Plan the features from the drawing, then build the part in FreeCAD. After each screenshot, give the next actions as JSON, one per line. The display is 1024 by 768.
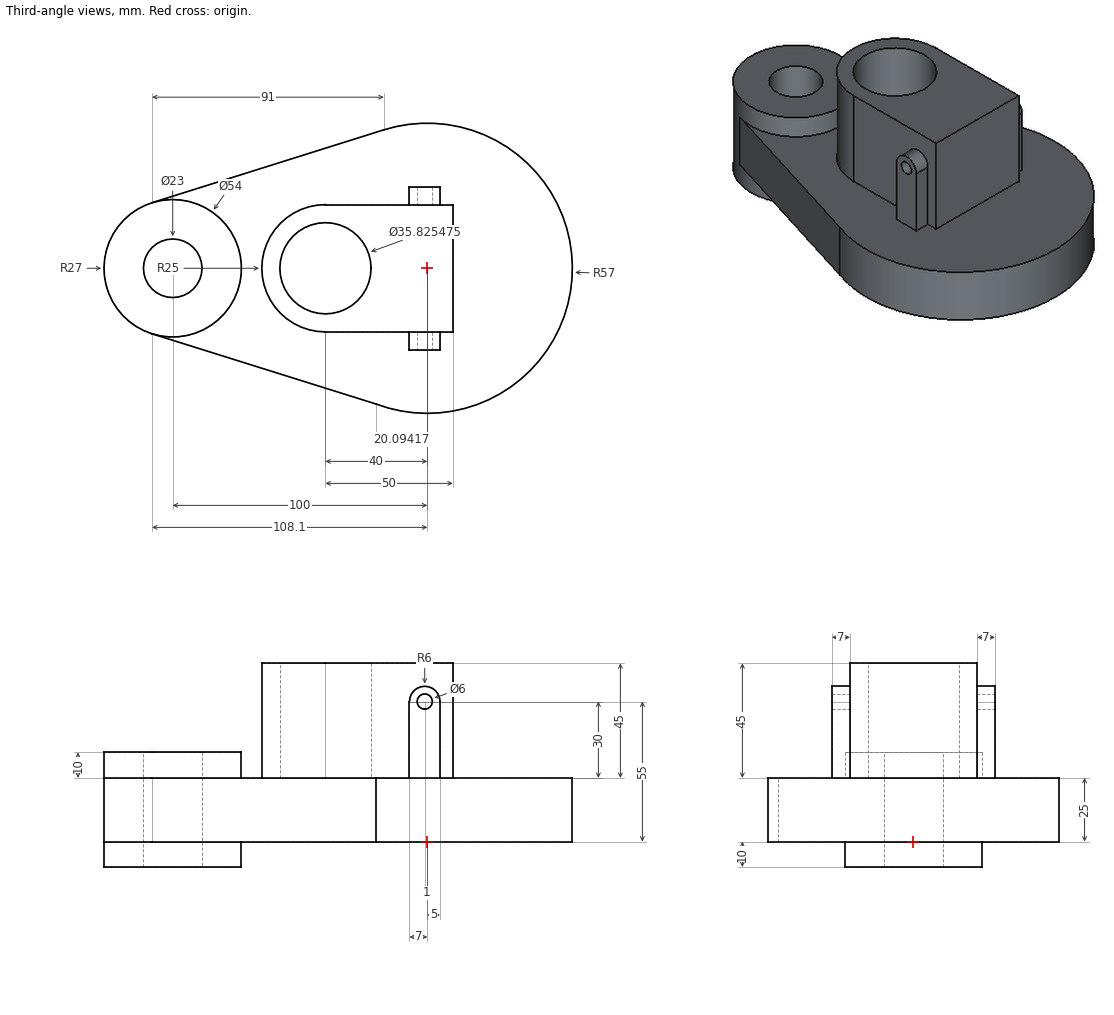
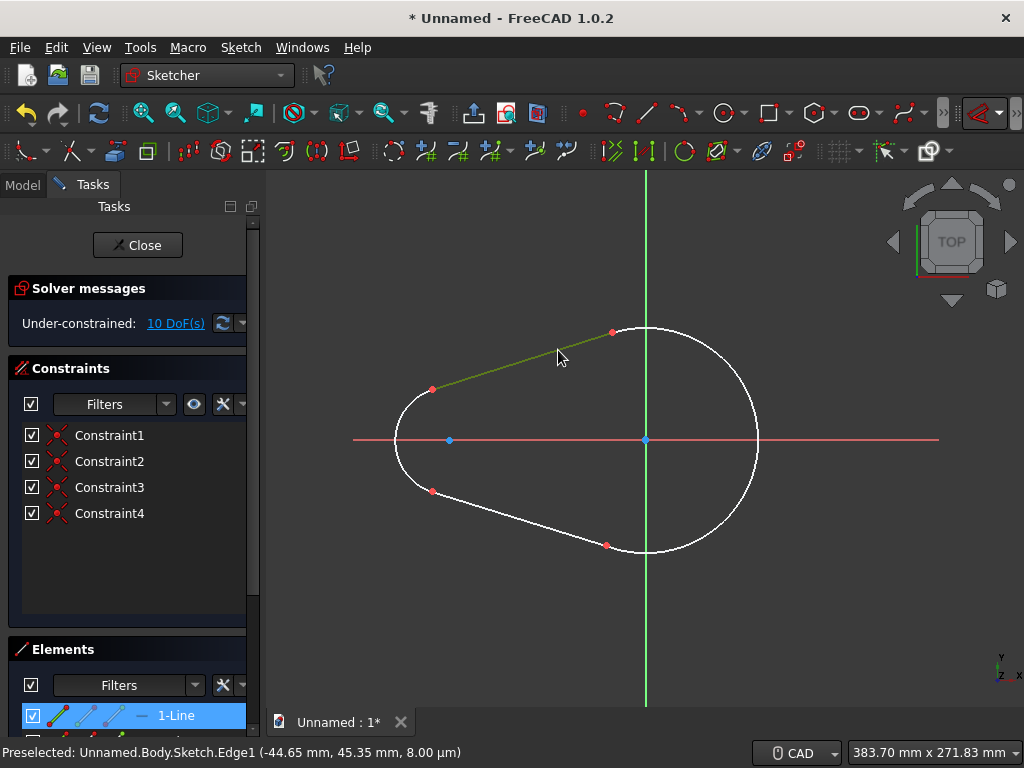
{"action": "left_click", "coordinate": [402, 415]}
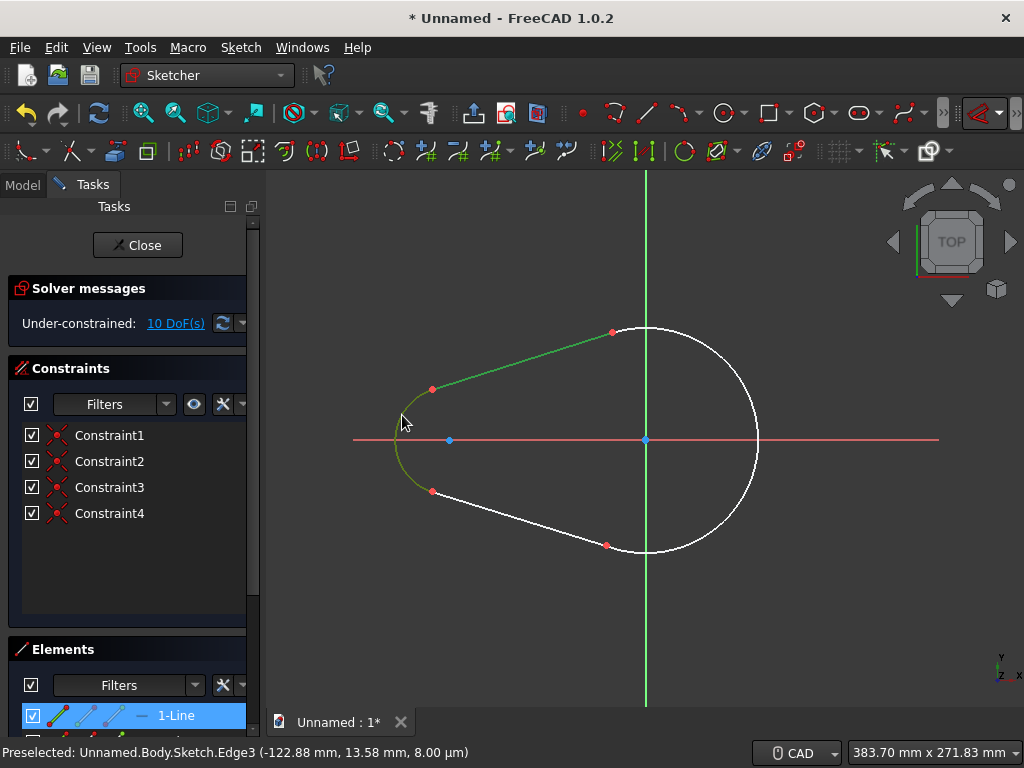
{"action": "key", "text": "t"}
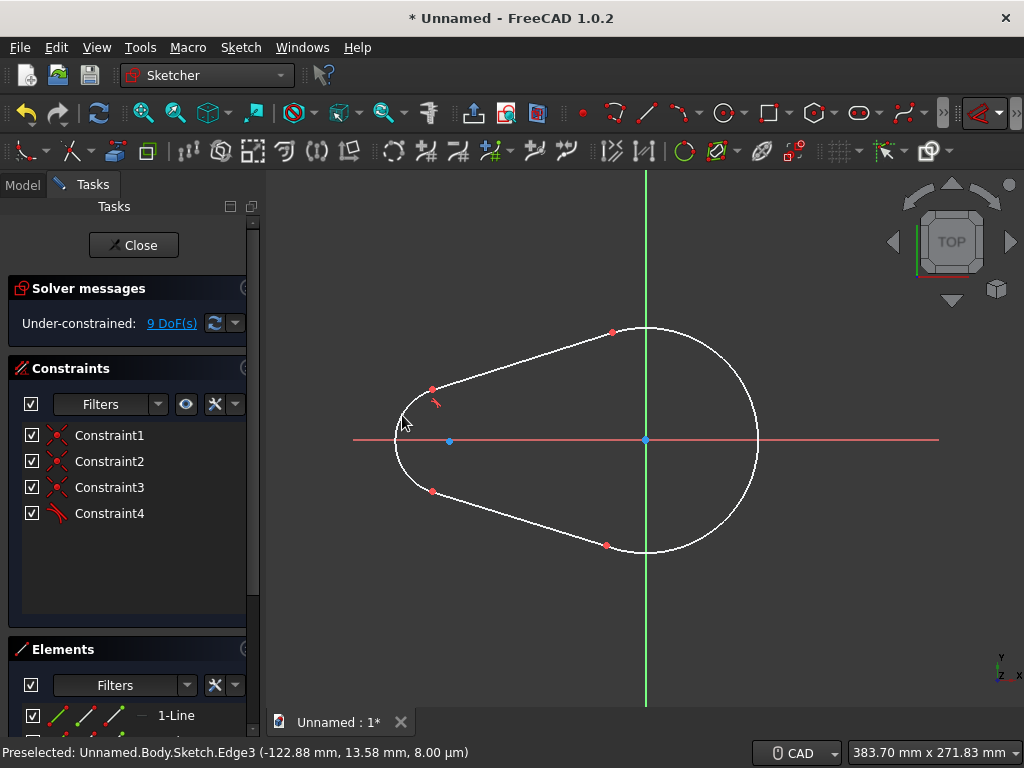
{"action": "left_click_drag", "start_coordinate": [636, 430], "coordinate": [656, 451]}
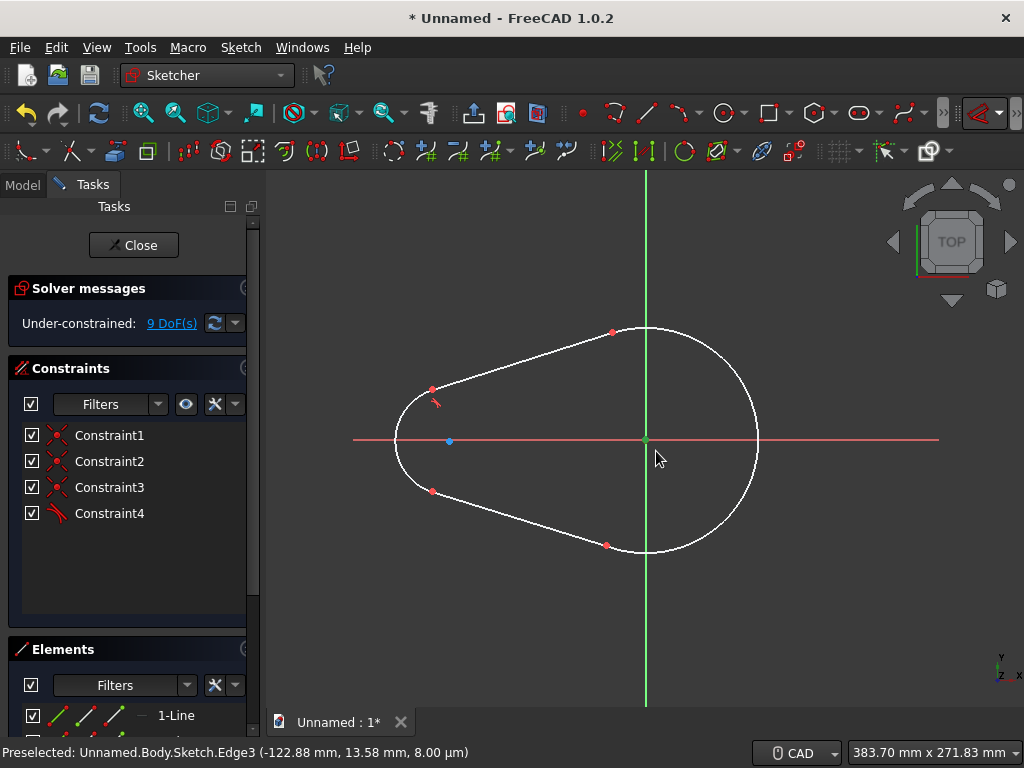
{"action": "key", "text": "c"}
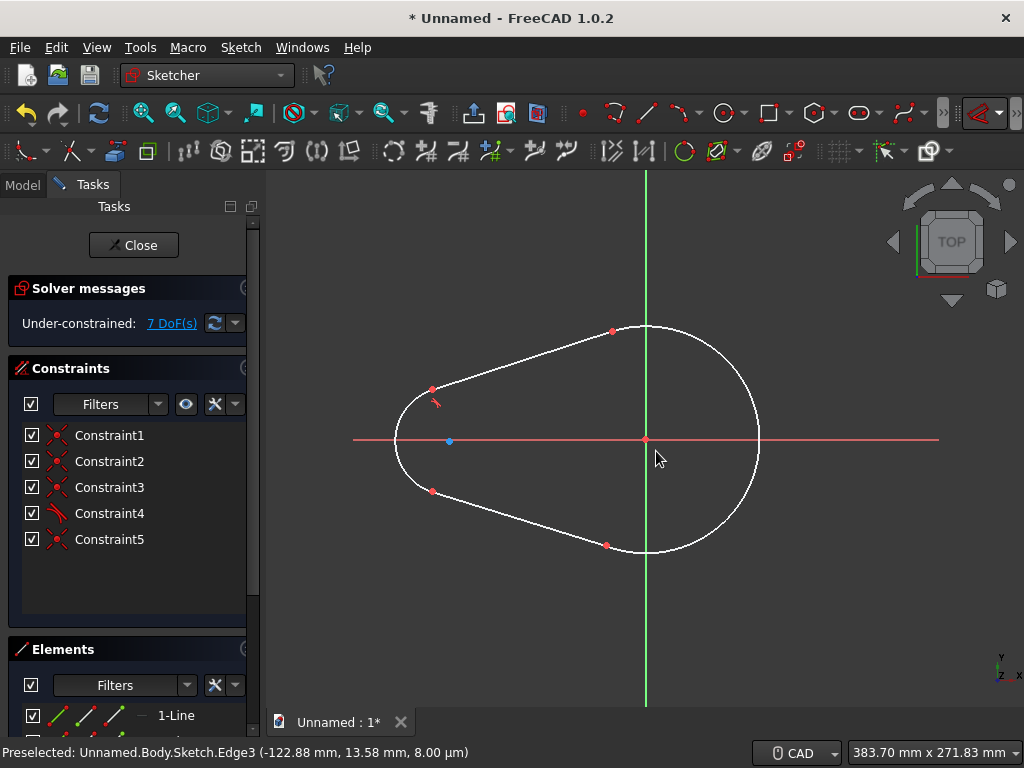
{"action": "left_click", "coordinate": [449, 441]}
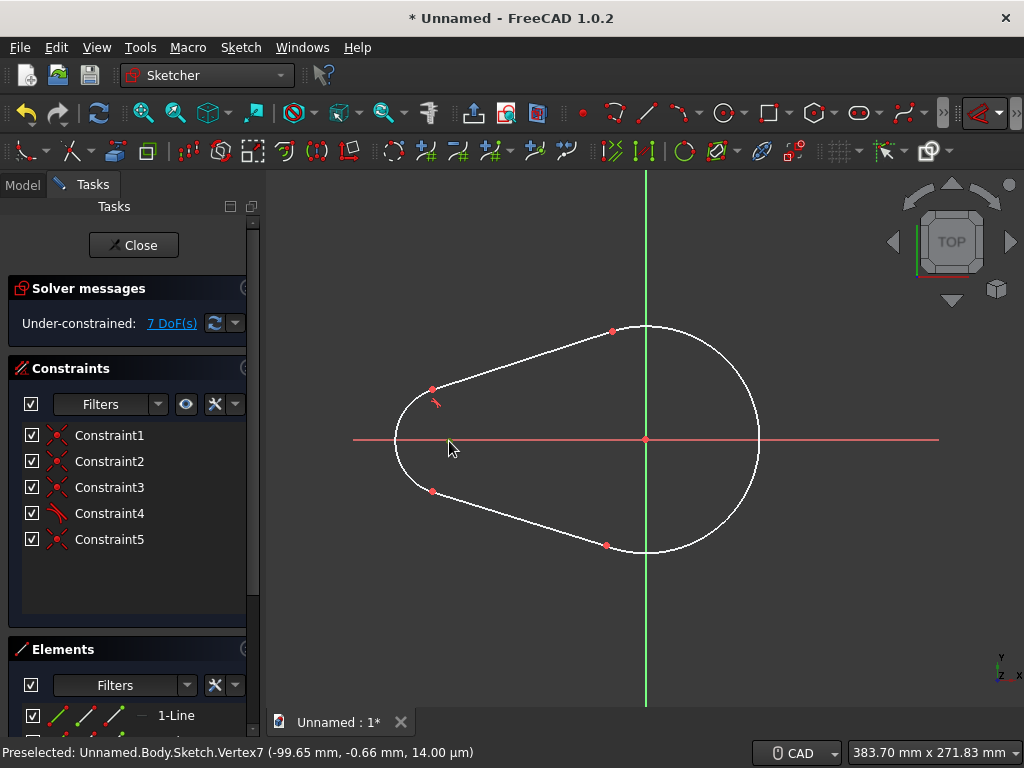
{"action": "left_click", "coordinate": [455, 440]}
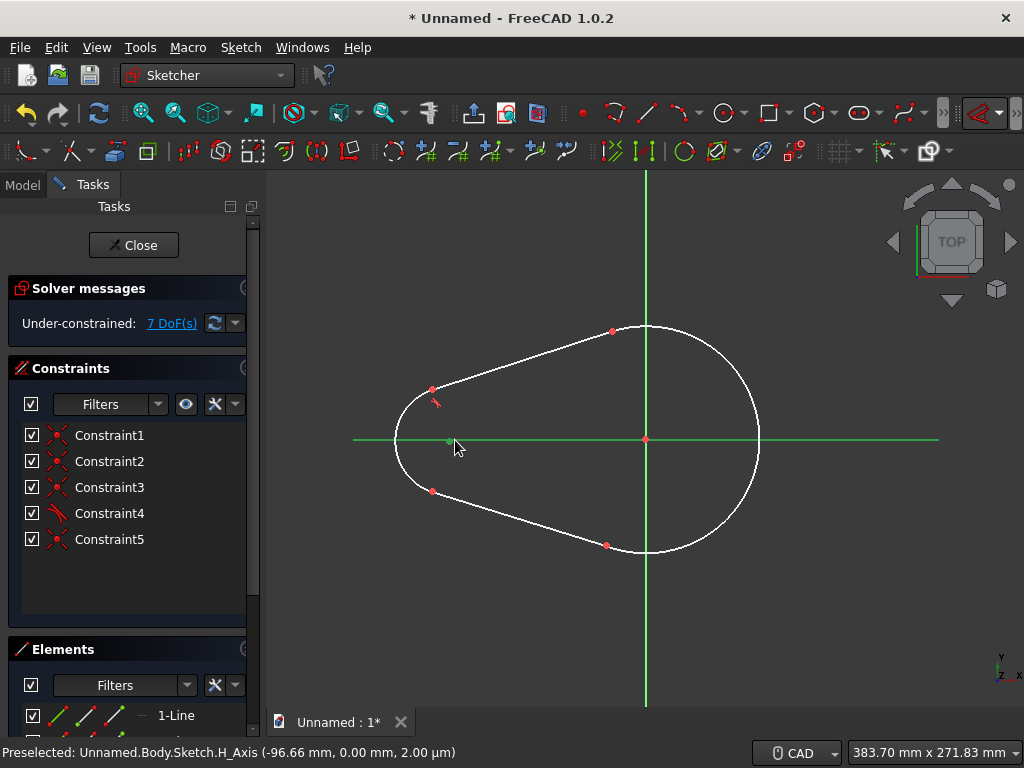
{"action": "key", "text": "c"}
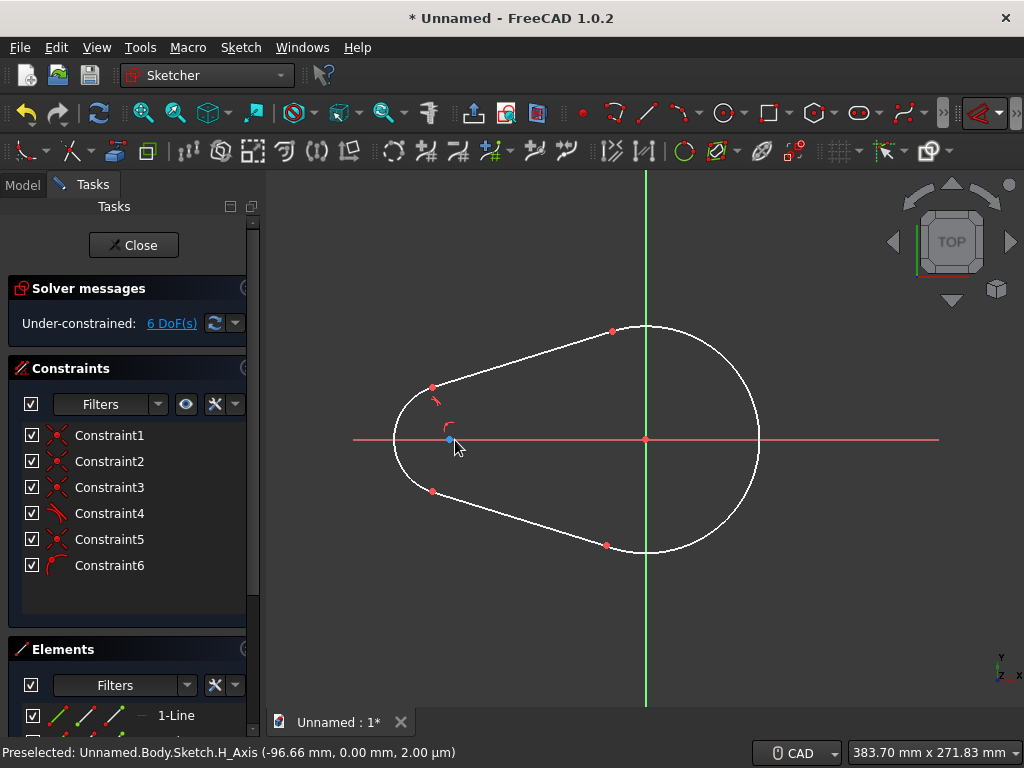
{"action": "left_click", "coordinate": [978, 114]}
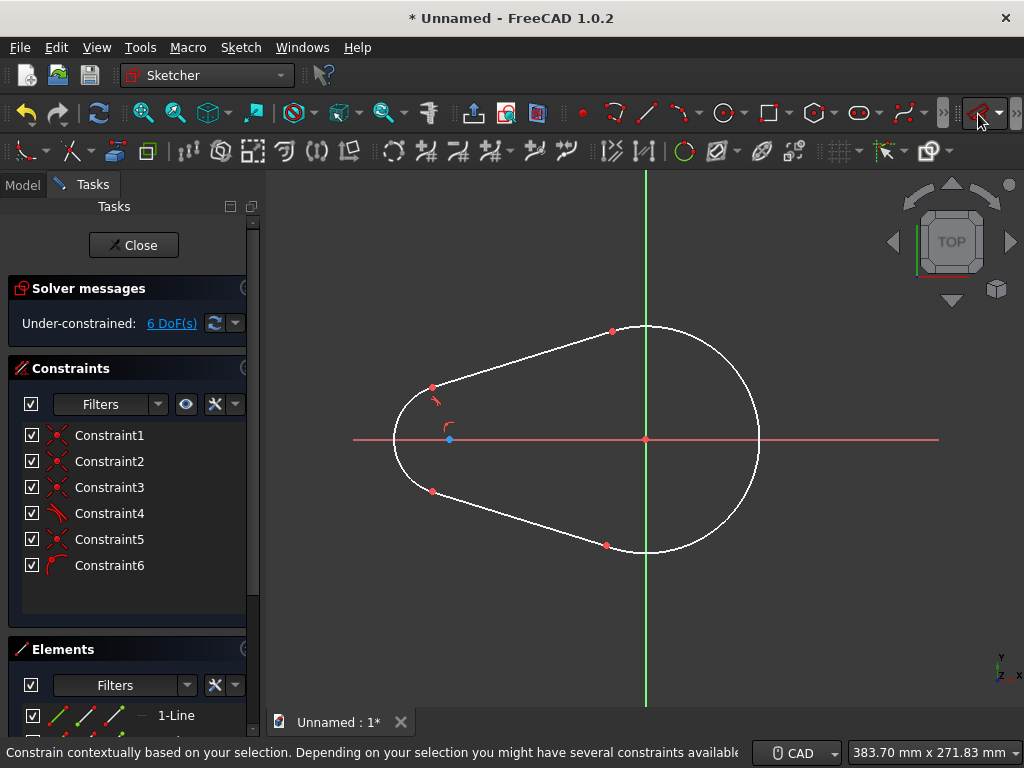
{"action": "left_click", "coordinate": [401, 413]}
{"action": "left_click", "coordinate": [373, 397]}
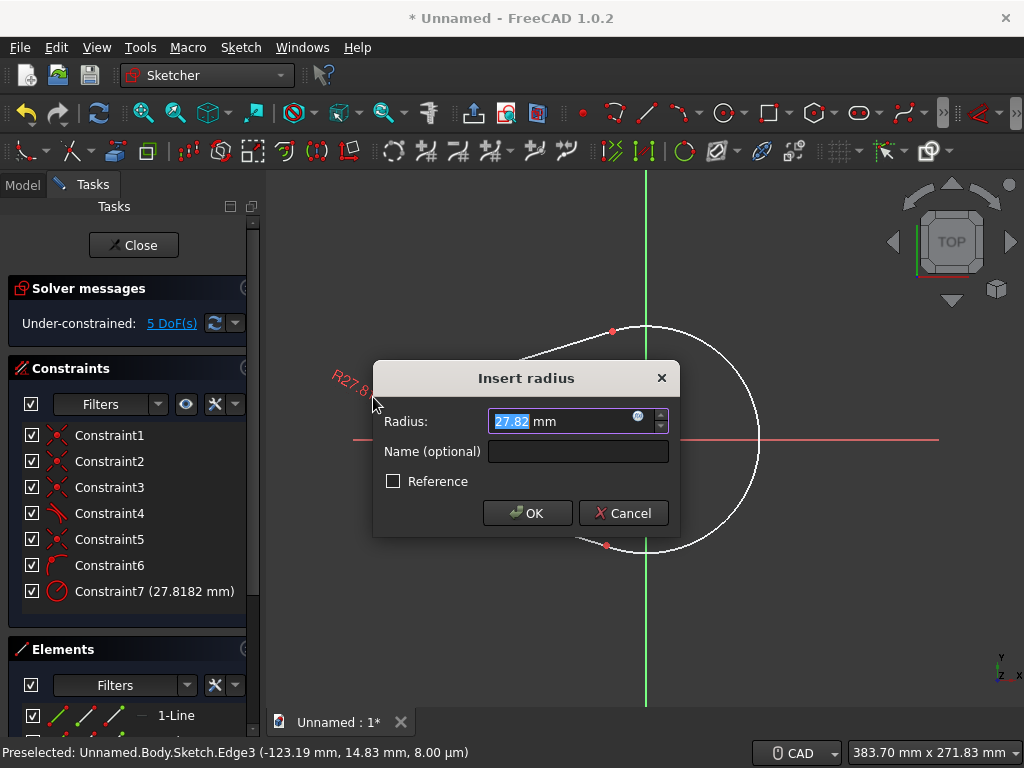
{"action": "type", "text": "27"}
{"action": "key", "text": "Return"}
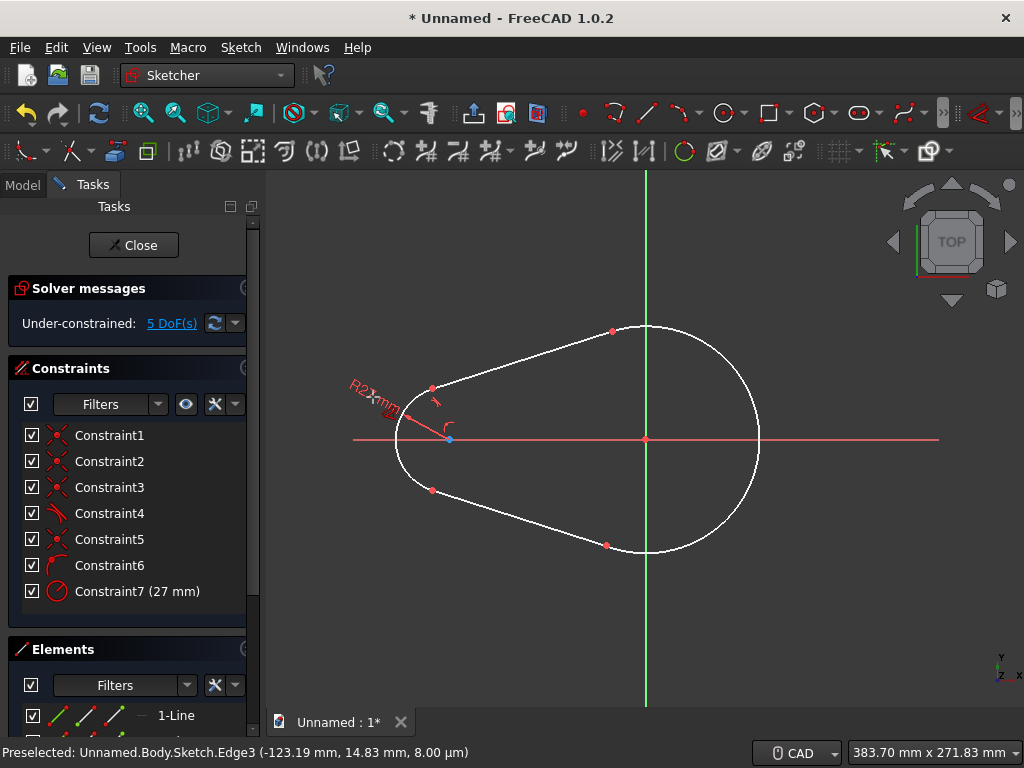
{"action": "left_click", "coordinate": [726, 520]}
{"action": "left_click", "coordinate": [749, 543]}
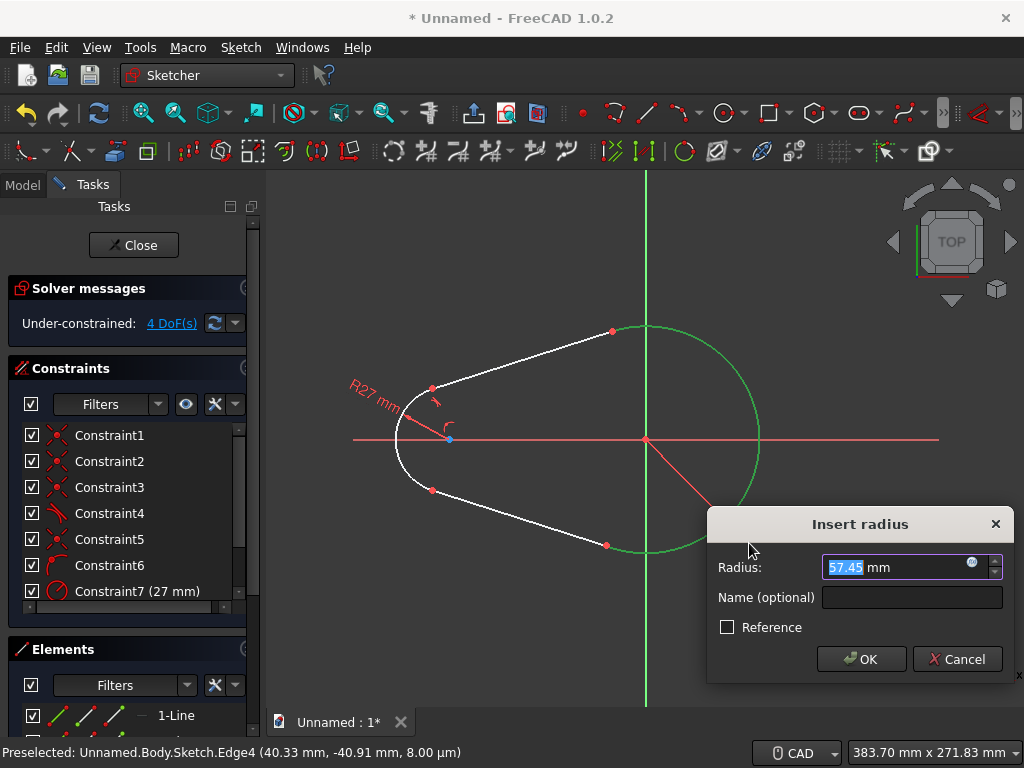
{"action": "type", "text": "57"}
{"action": "key", "text": "Return"}